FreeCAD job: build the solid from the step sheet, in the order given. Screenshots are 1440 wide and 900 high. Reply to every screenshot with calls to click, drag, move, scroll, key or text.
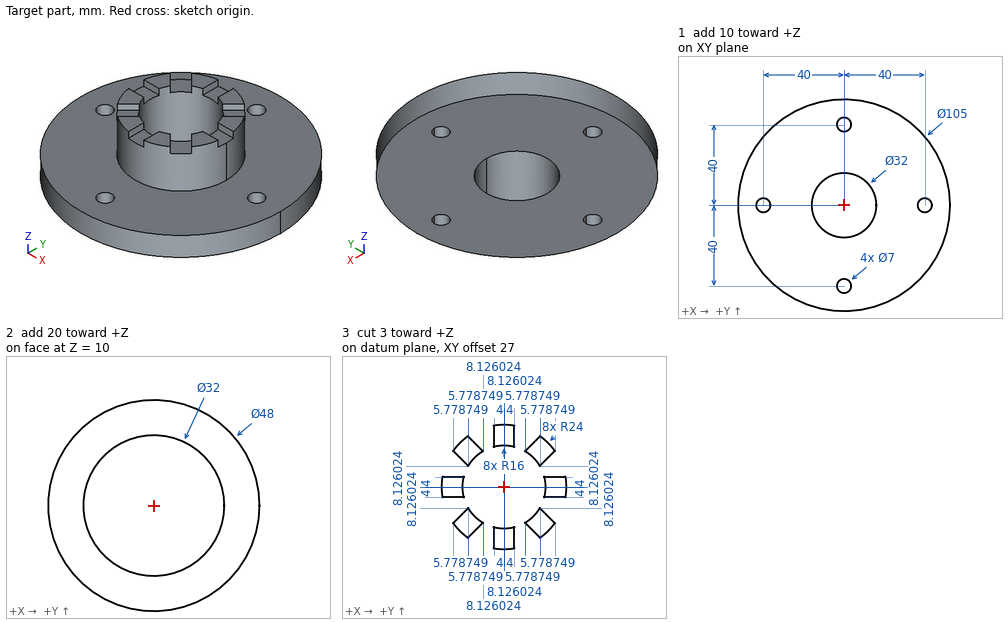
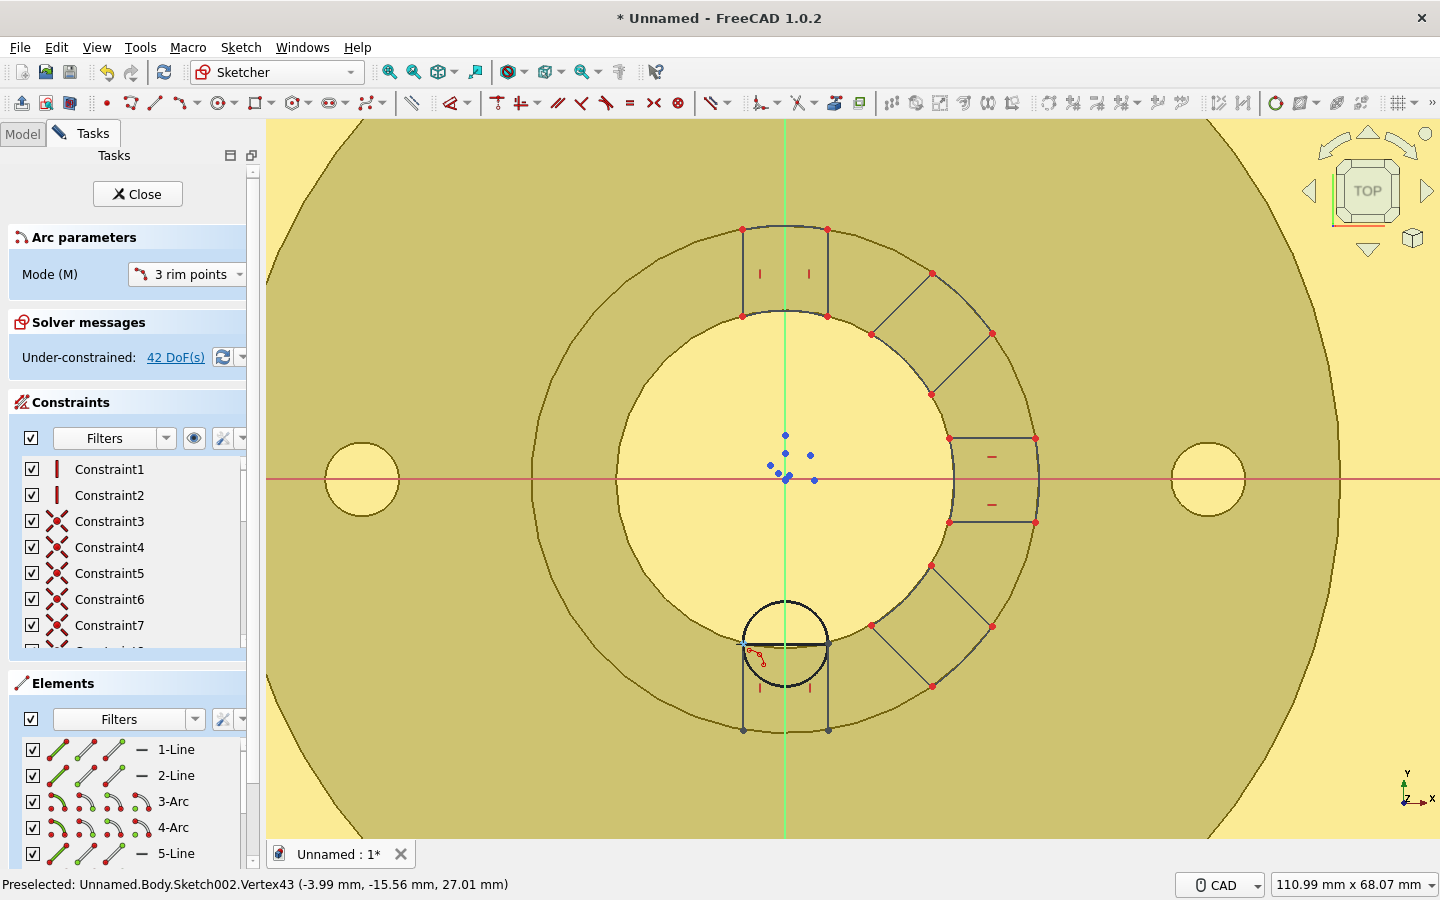
scroll(777, 648, up, 6)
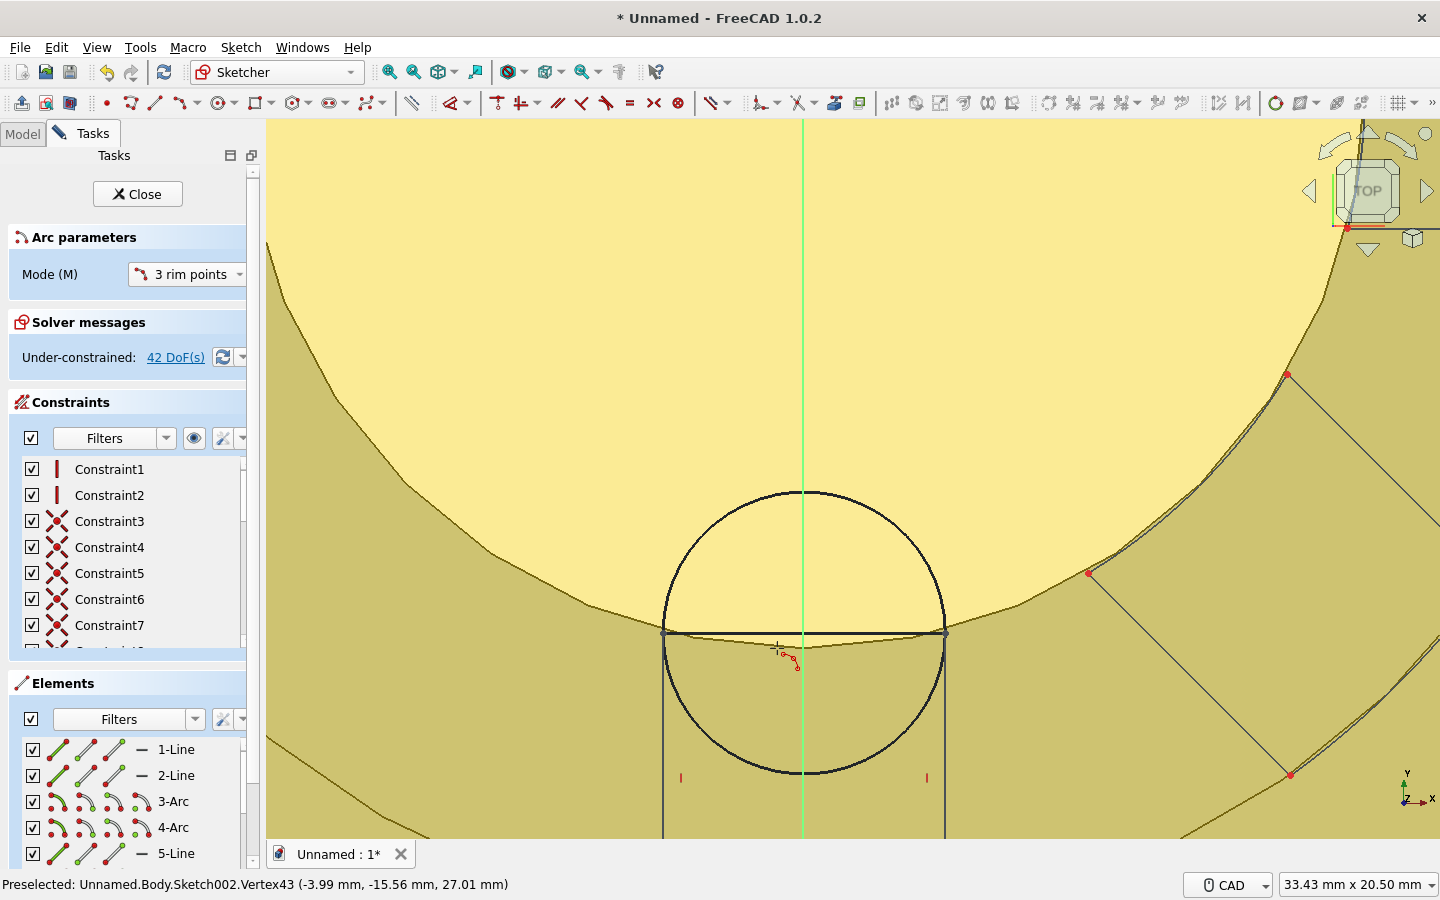
click(775, 648)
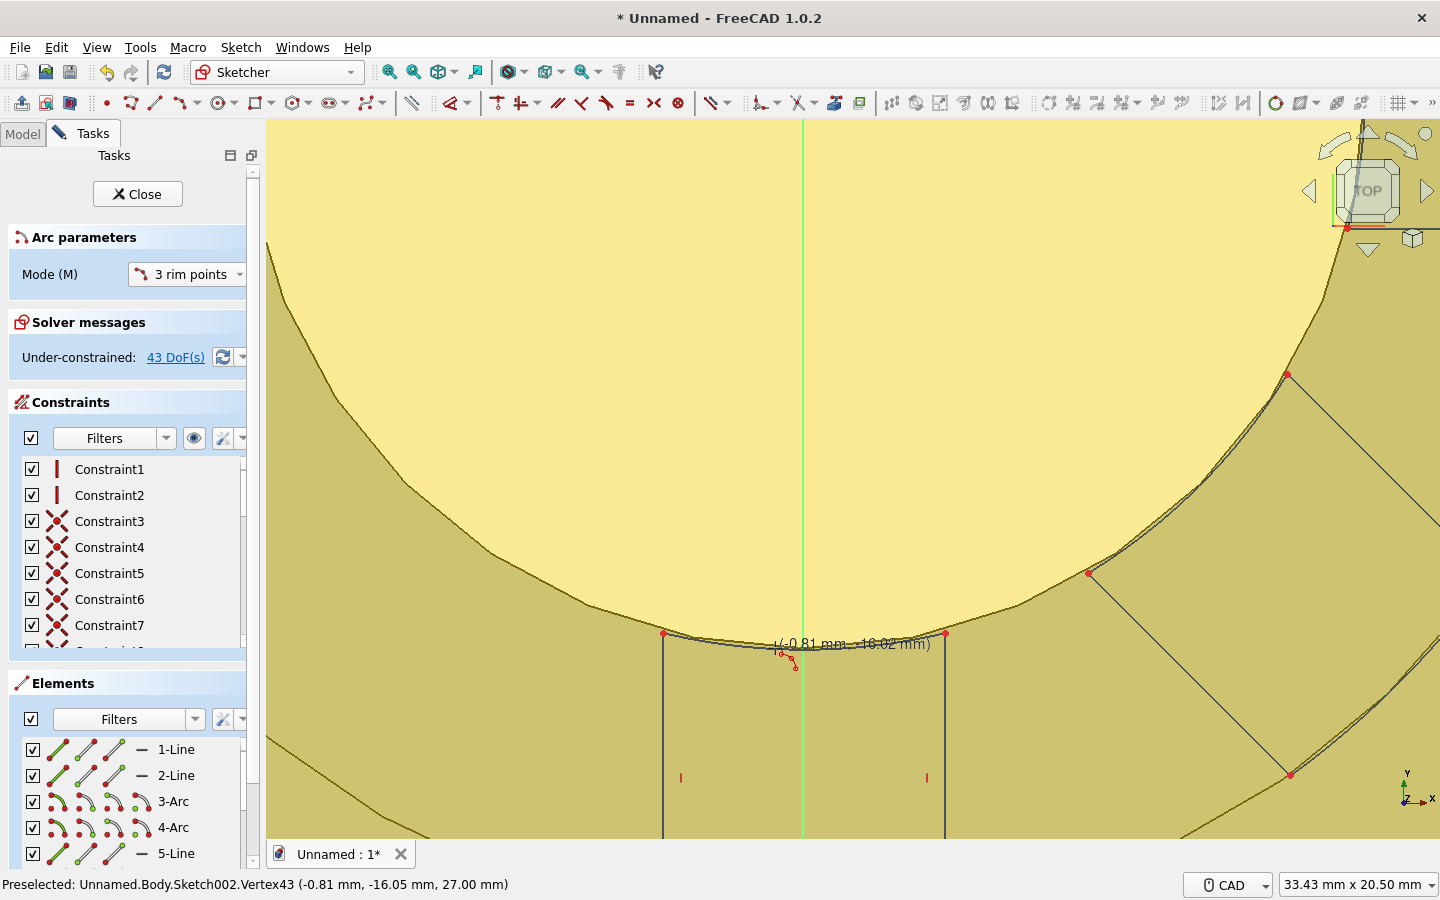
scroll(776, 648, down, 6)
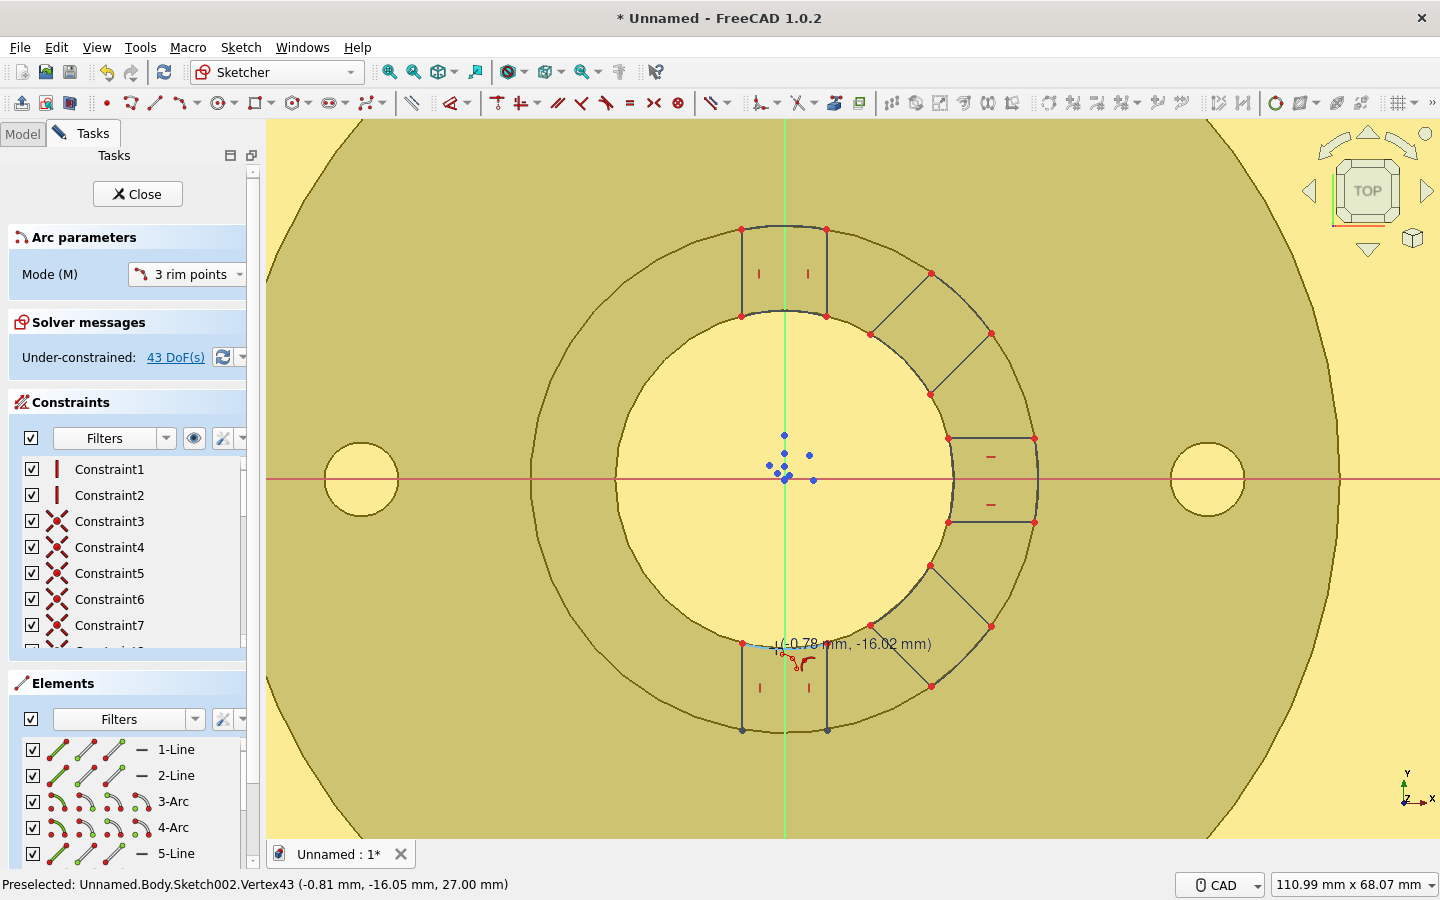
click(742, 731)
click(827, 731)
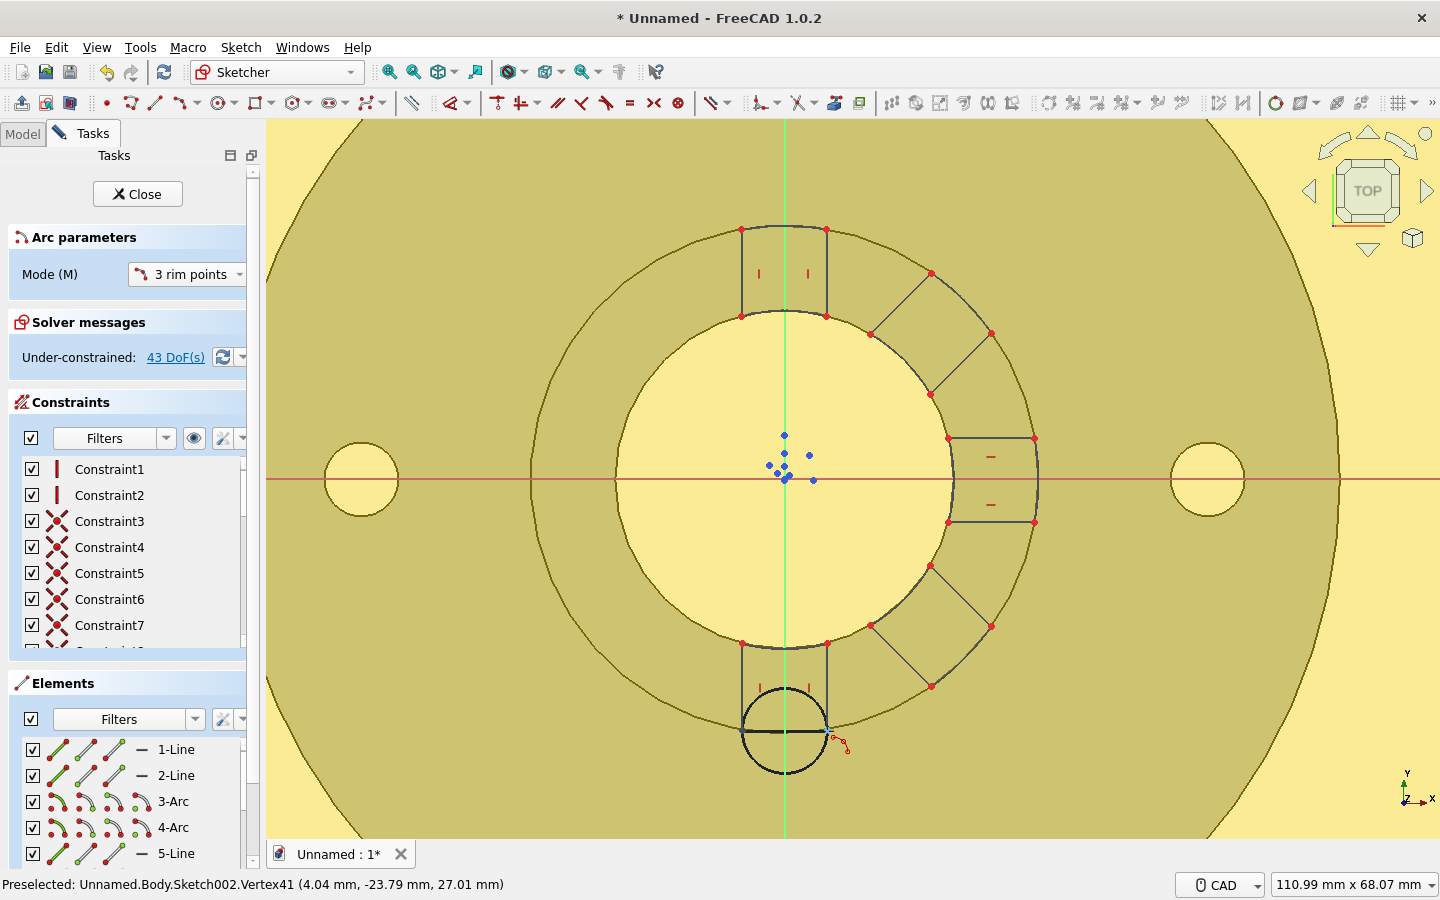
scroll(776, 733, up, 8)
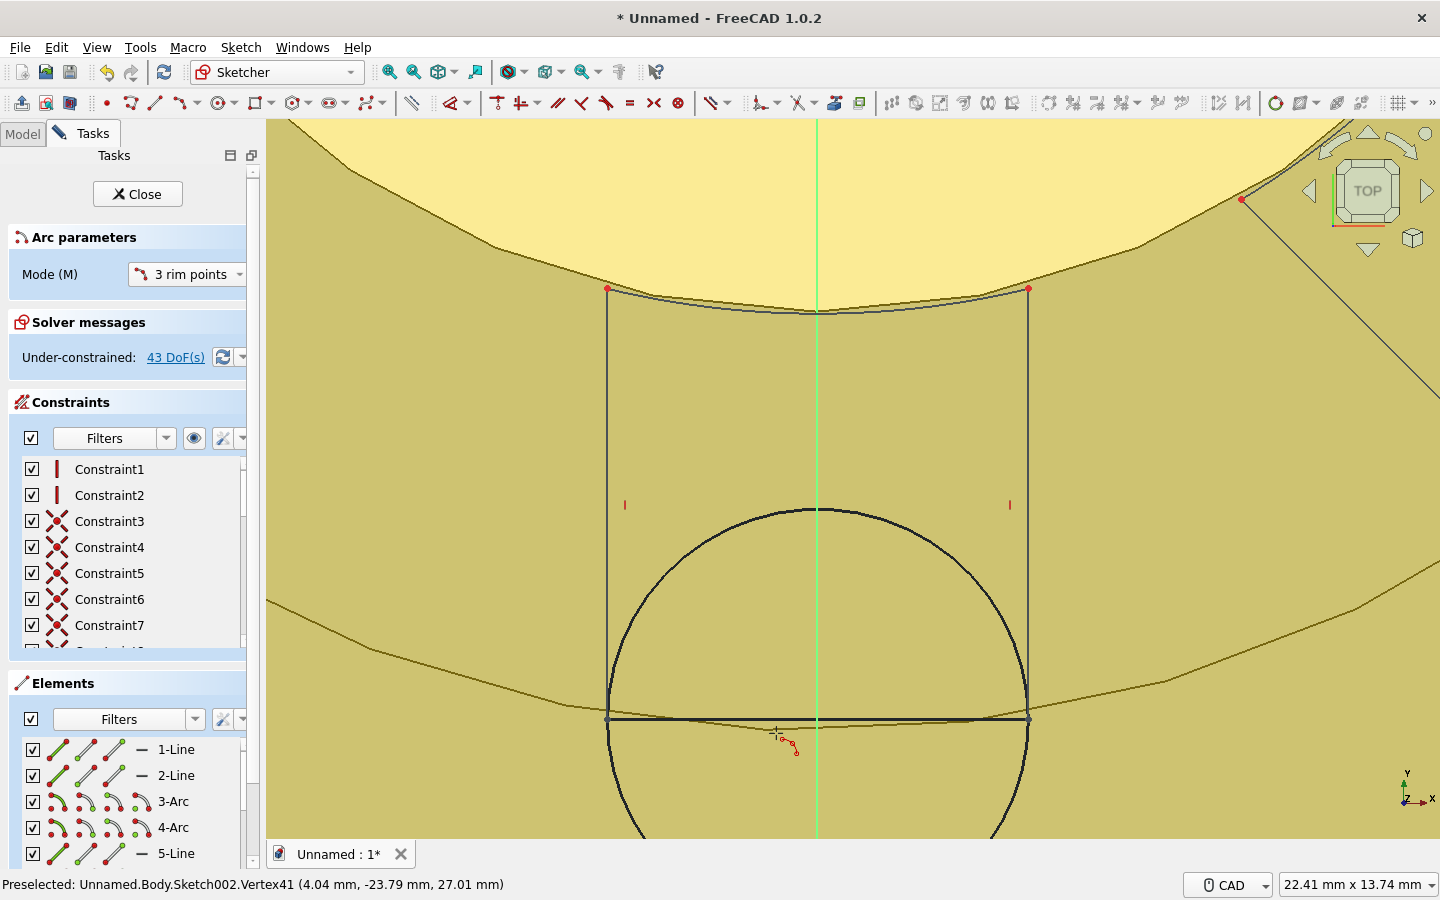
click(774, 730)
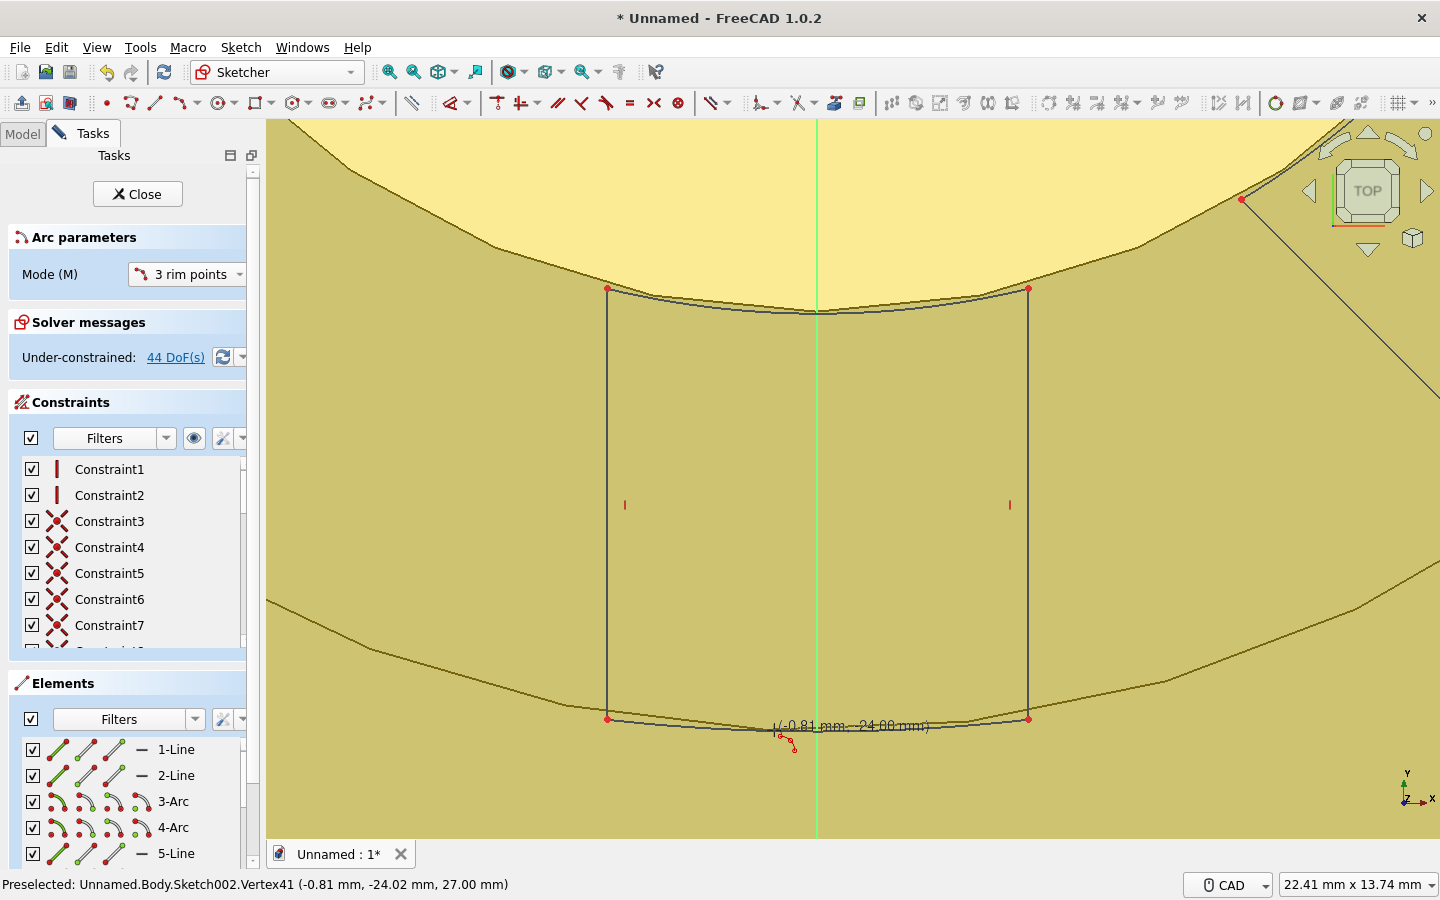
click(156, 104)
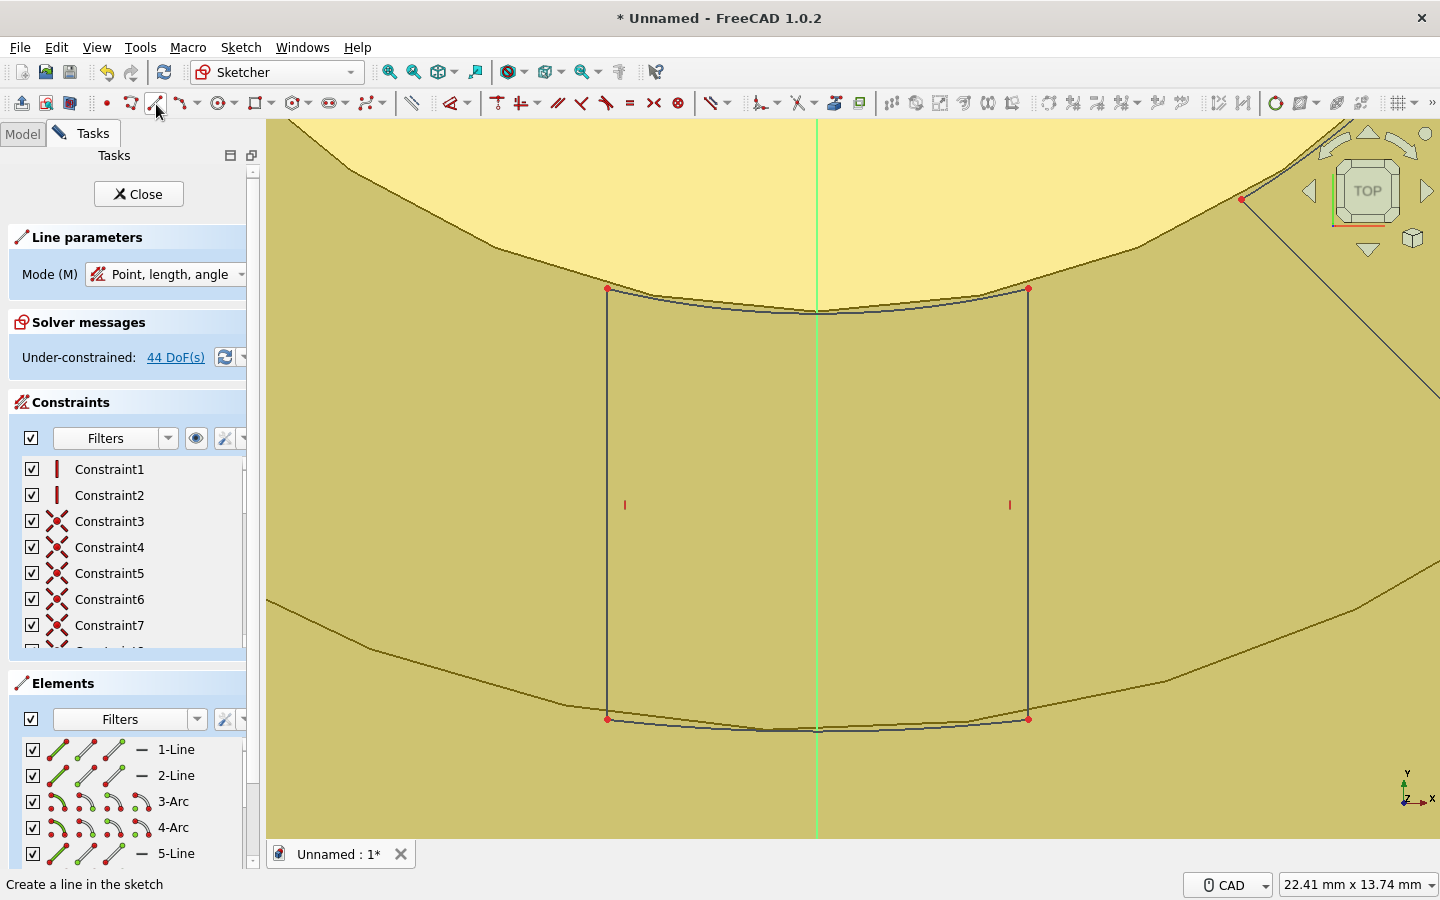
scroll(776, 733, down, 8)